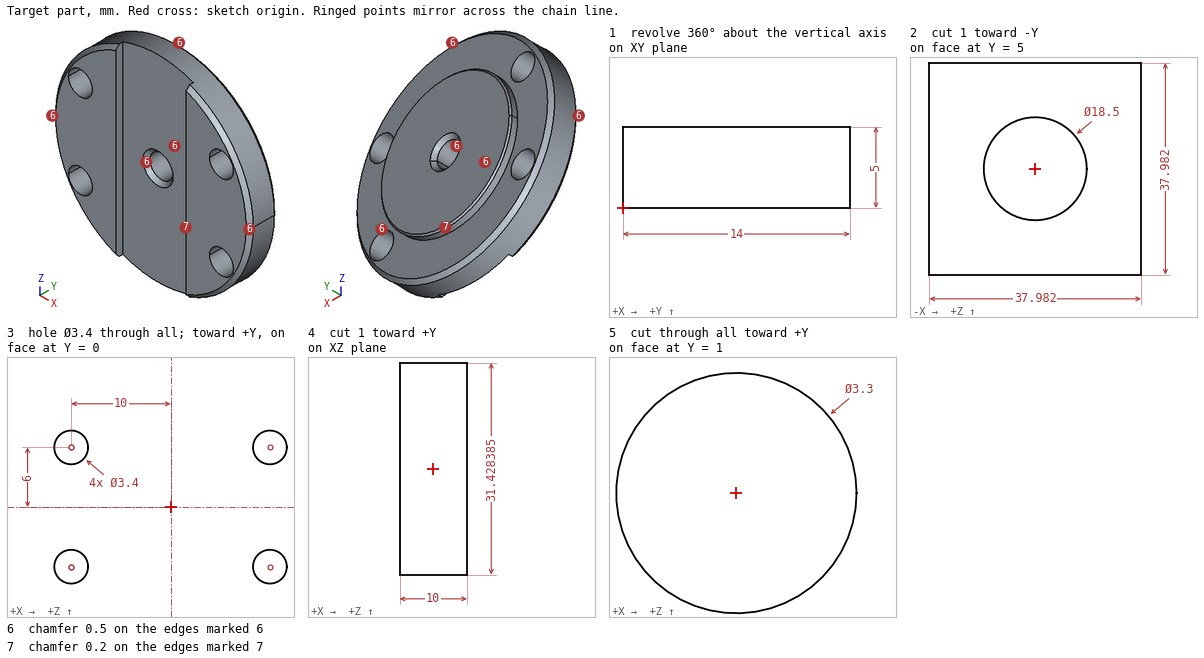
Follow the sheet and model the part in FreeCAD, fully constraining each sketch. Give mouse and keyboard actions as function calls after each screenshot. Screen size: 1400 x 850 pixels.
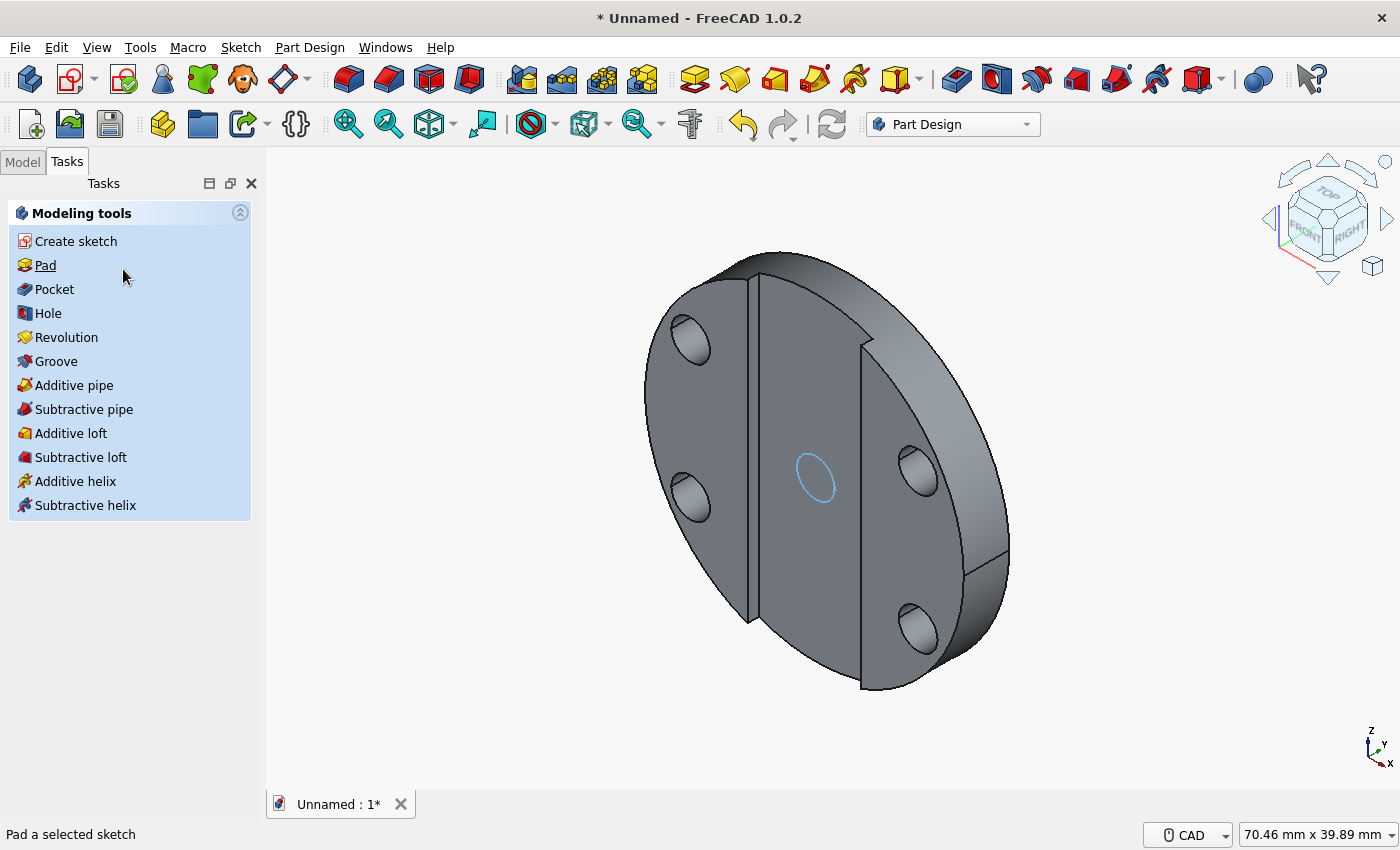
click(958, 80)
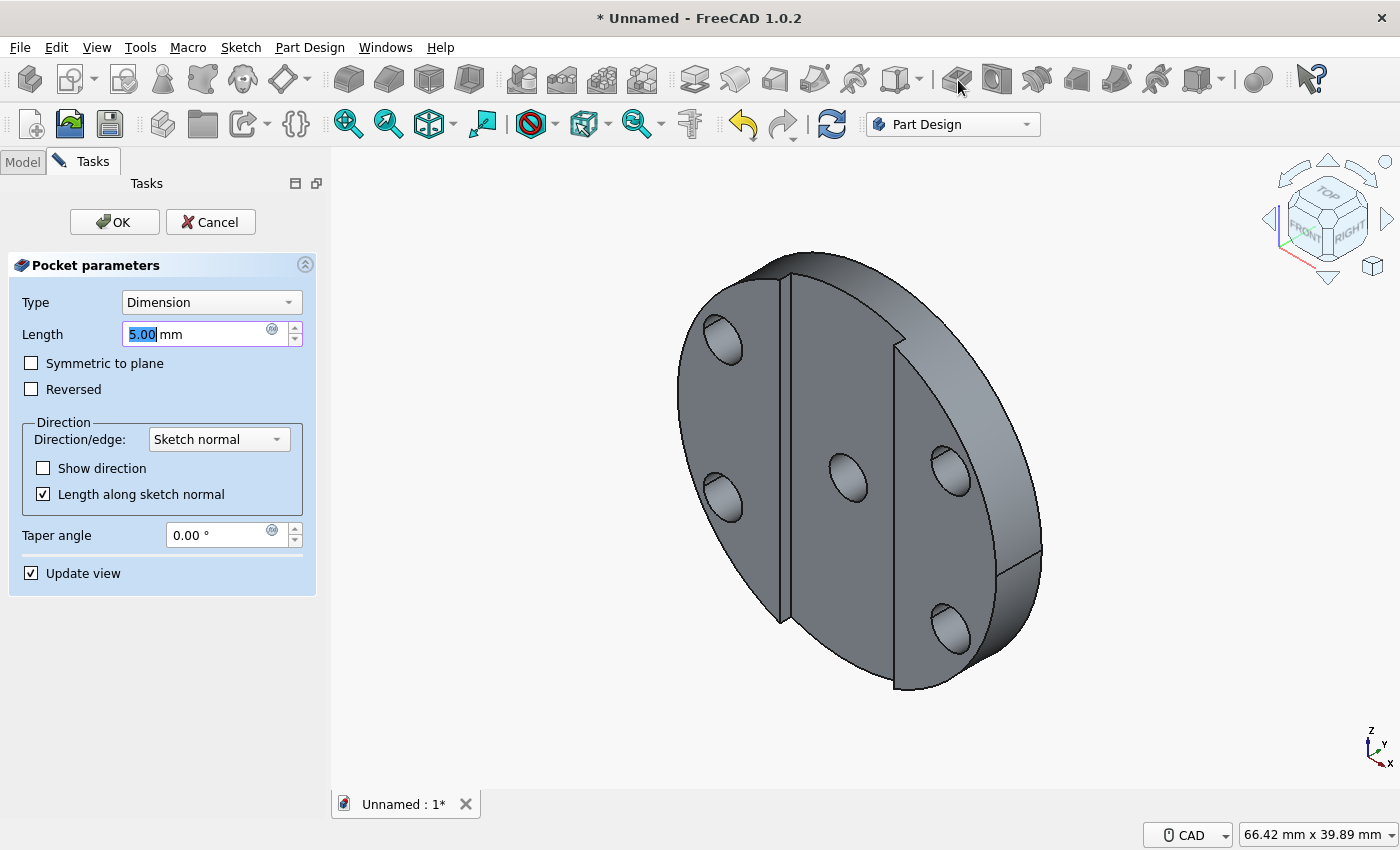
click(212, 302)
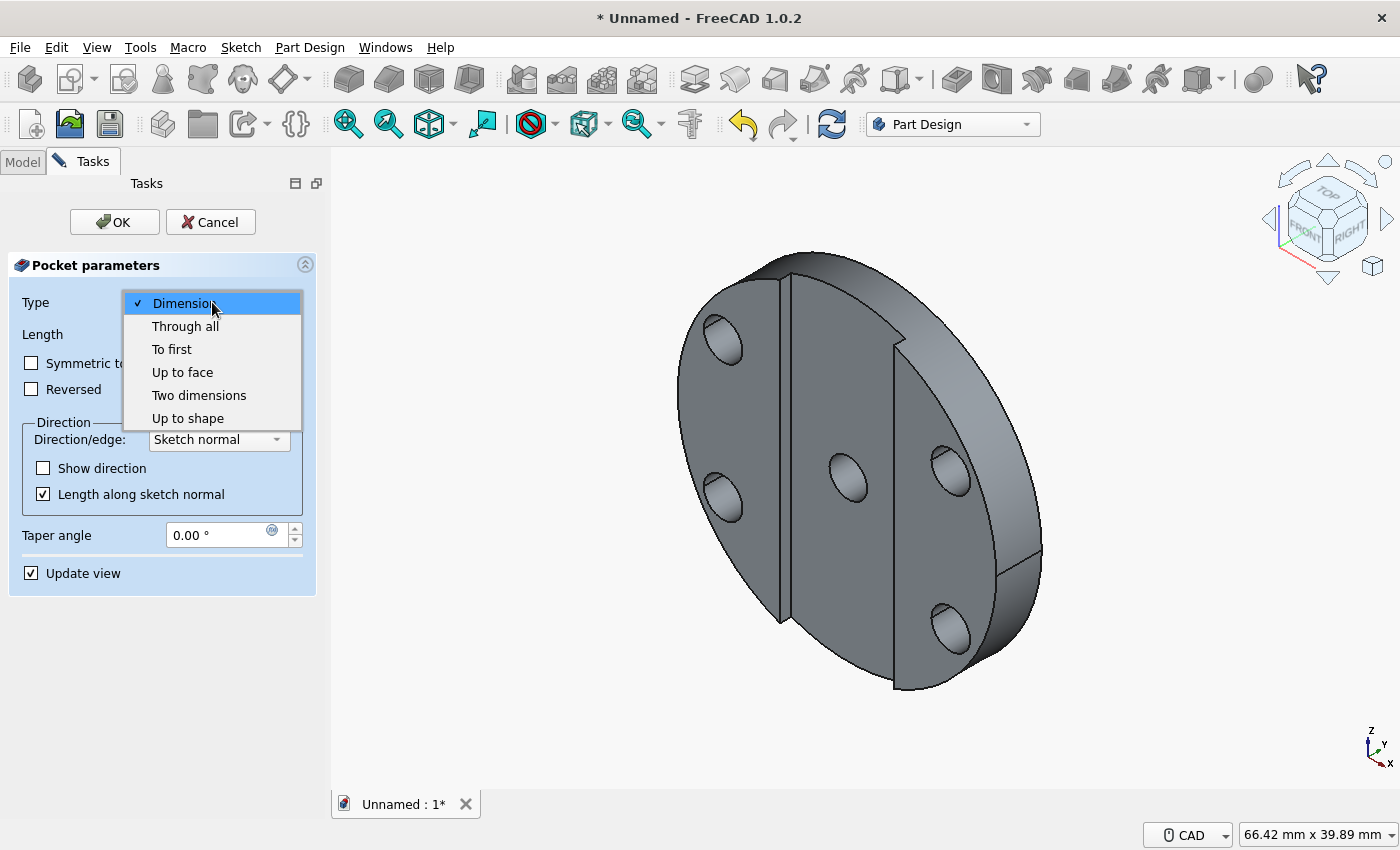
click(212, 326)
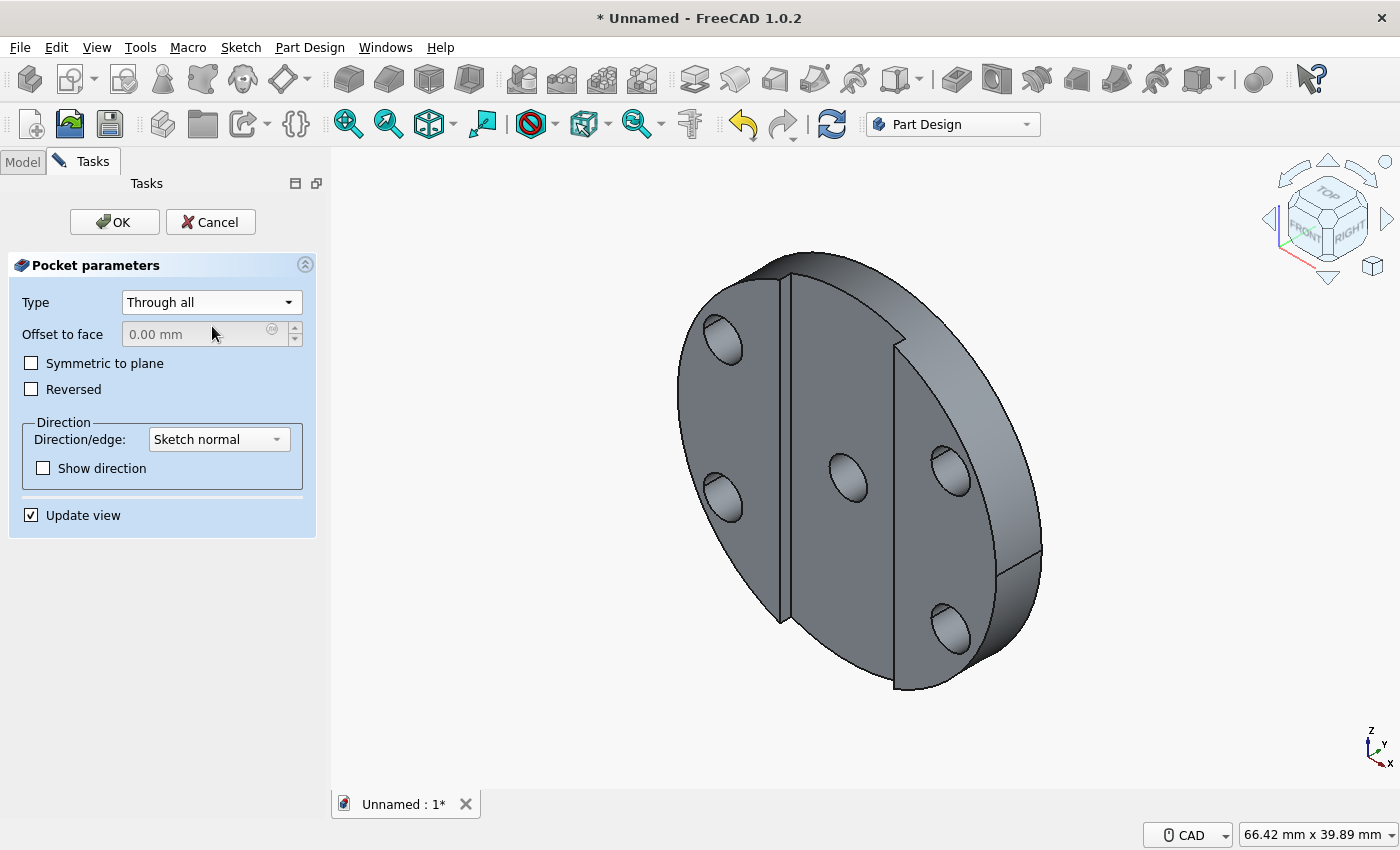
click(115, 222)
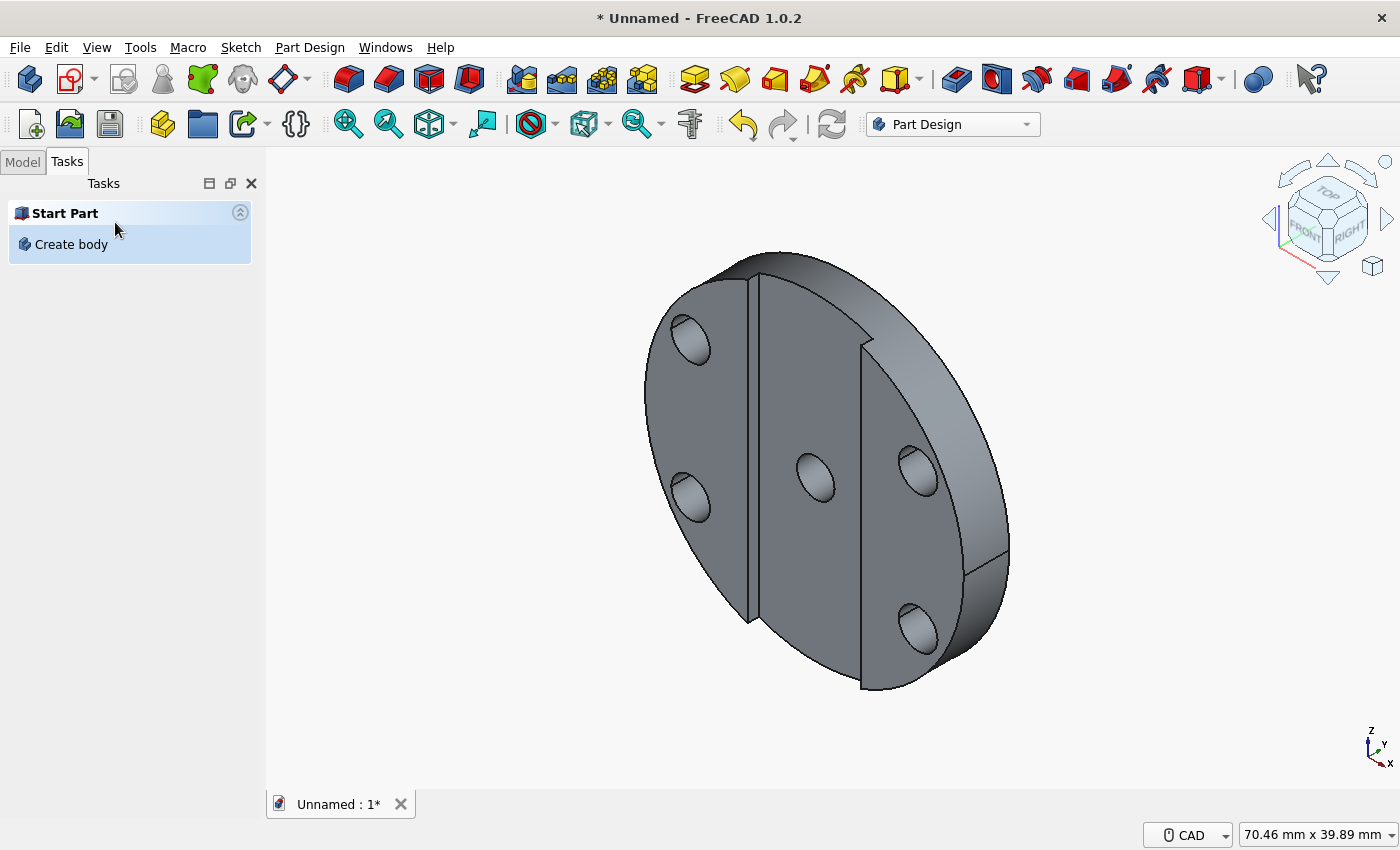
click(936, 455)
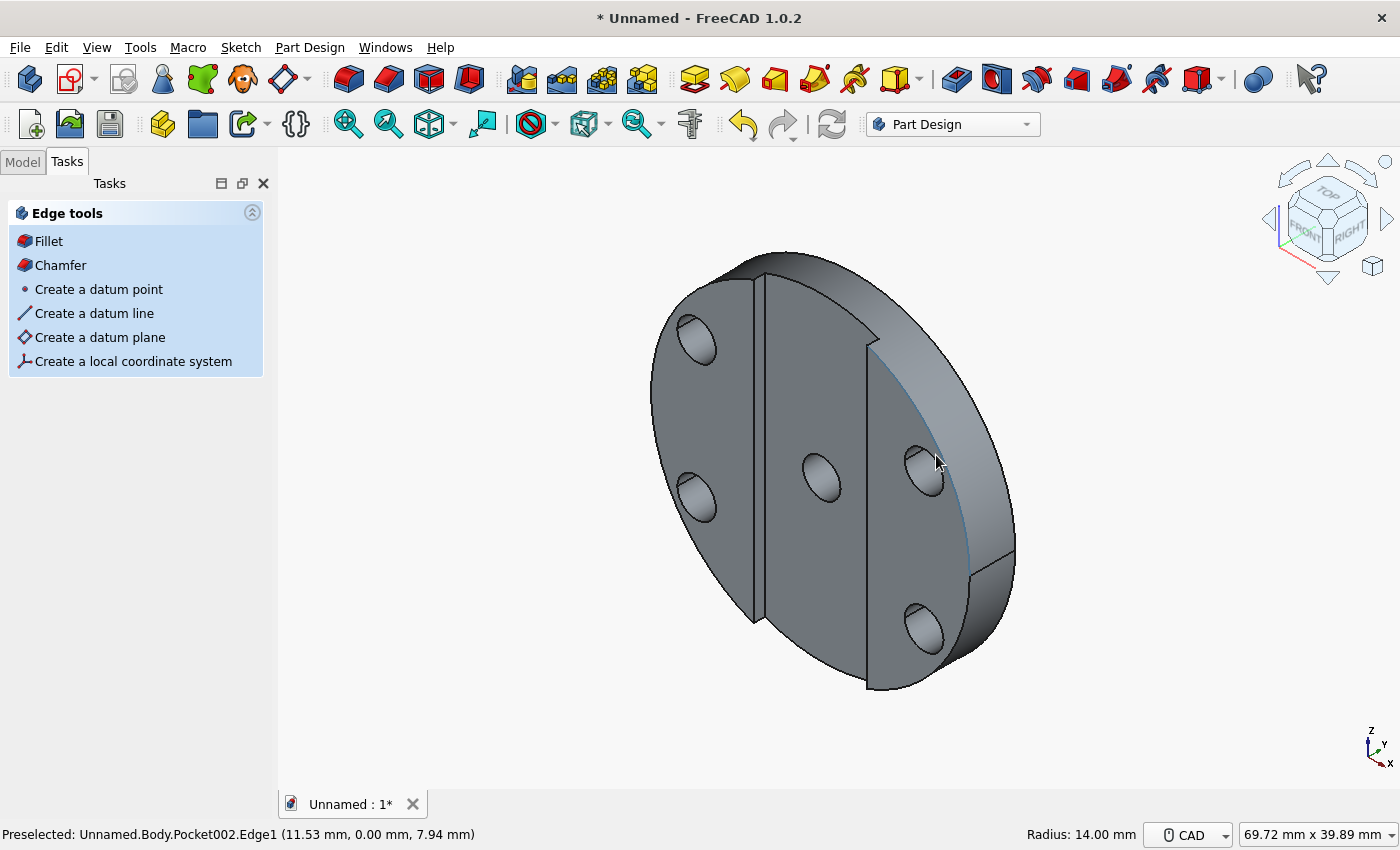
click(713, 281, ctrl)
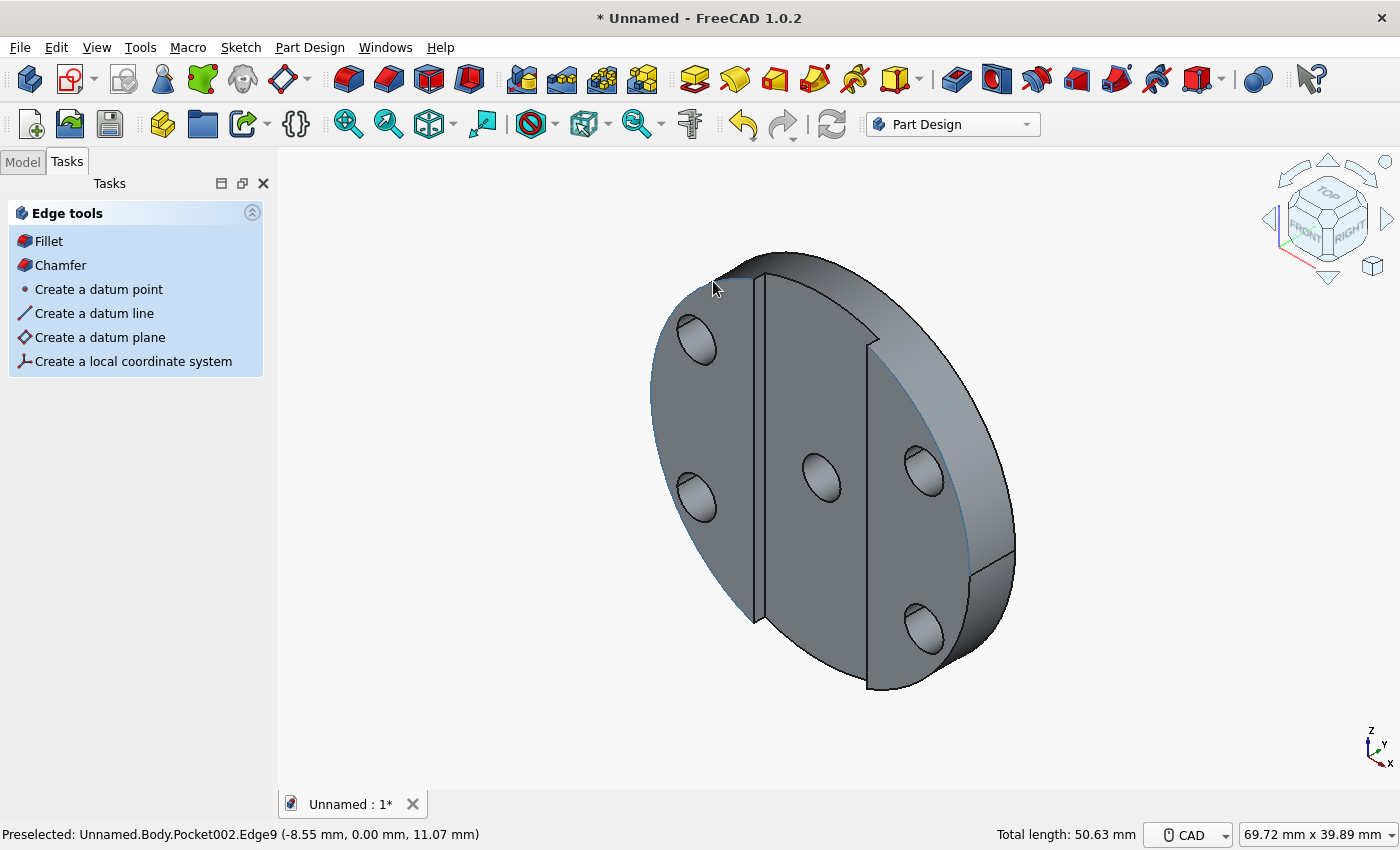
click(803, 466, ctrl)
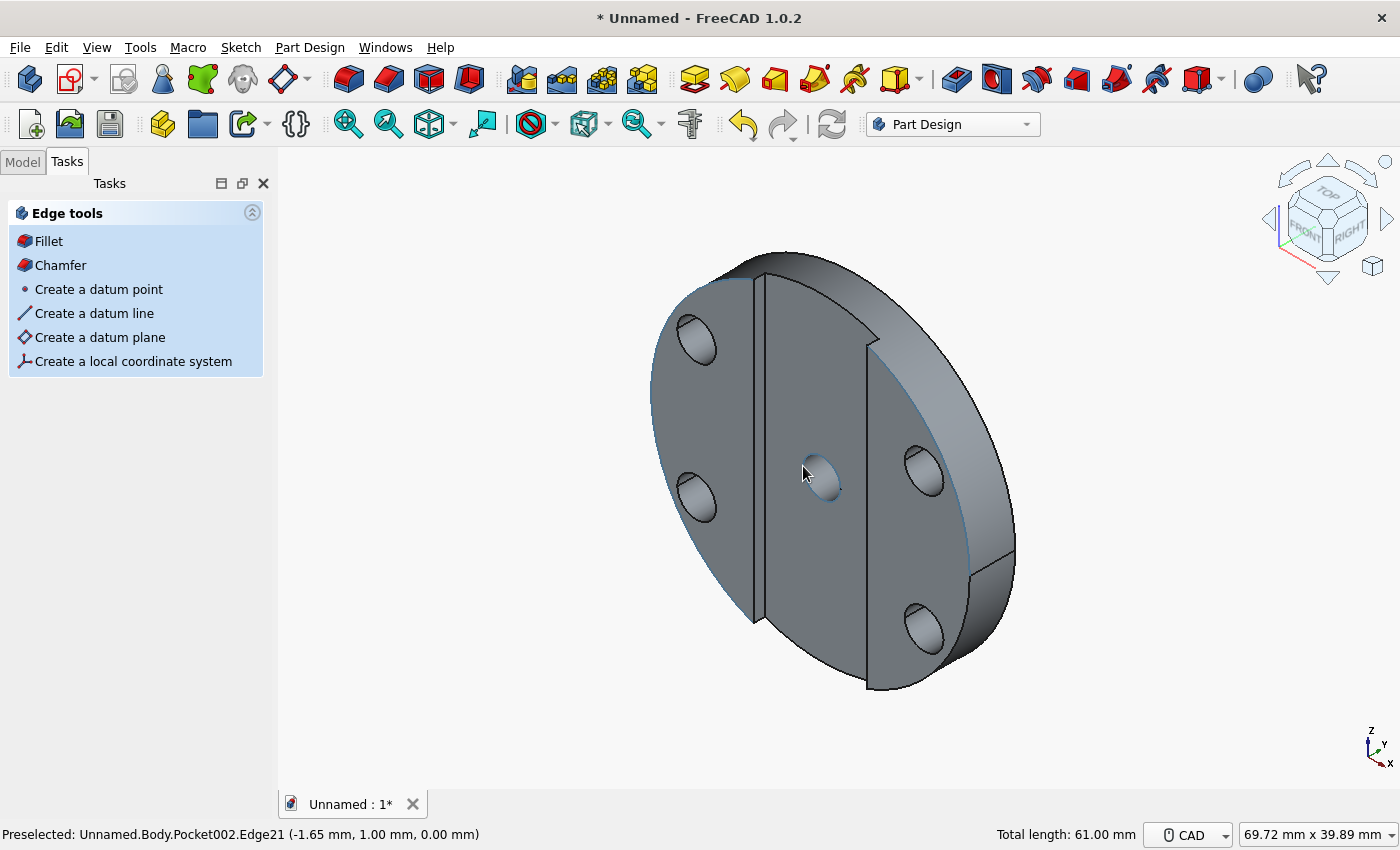
key(2)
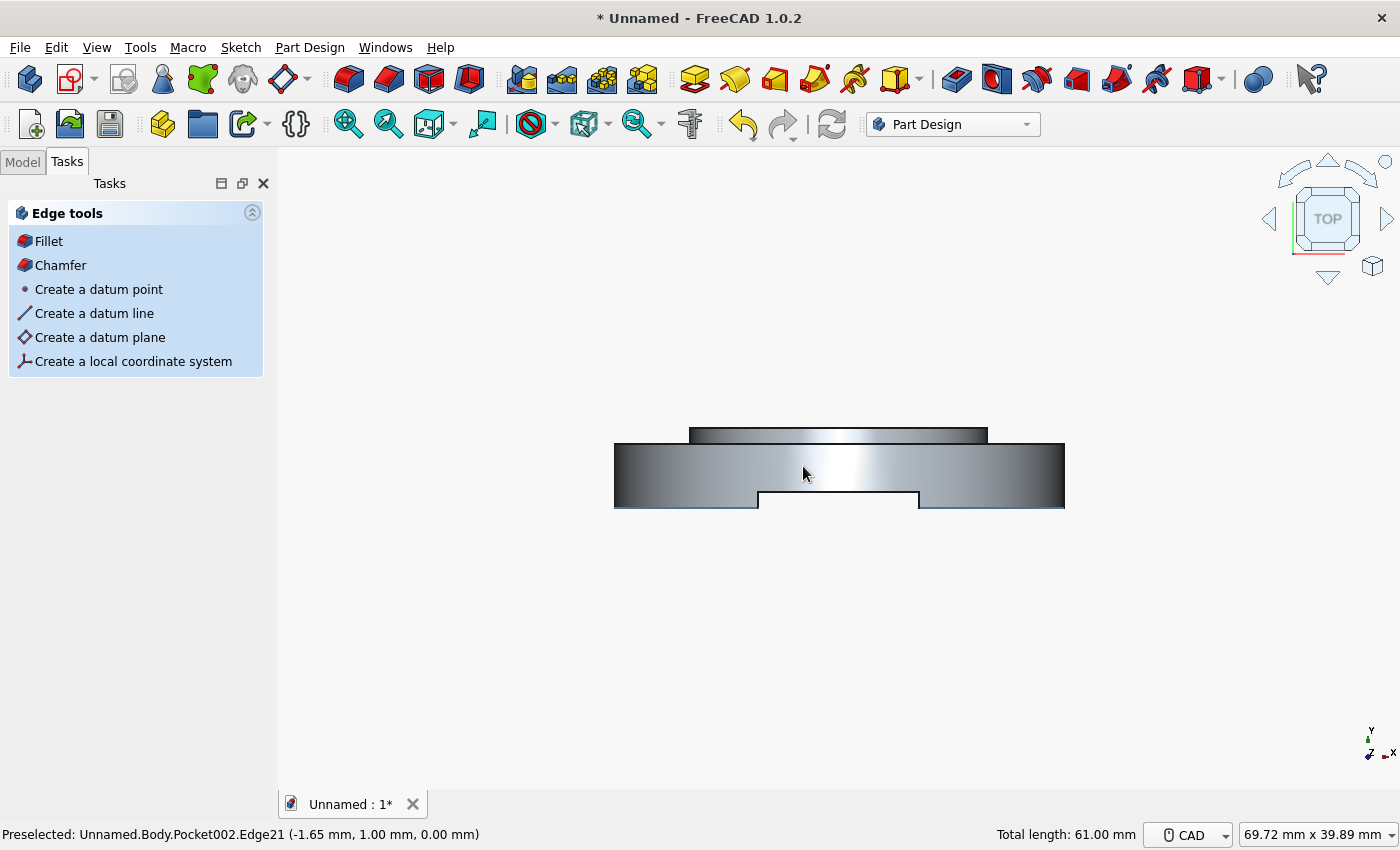
key(v)
key(f)